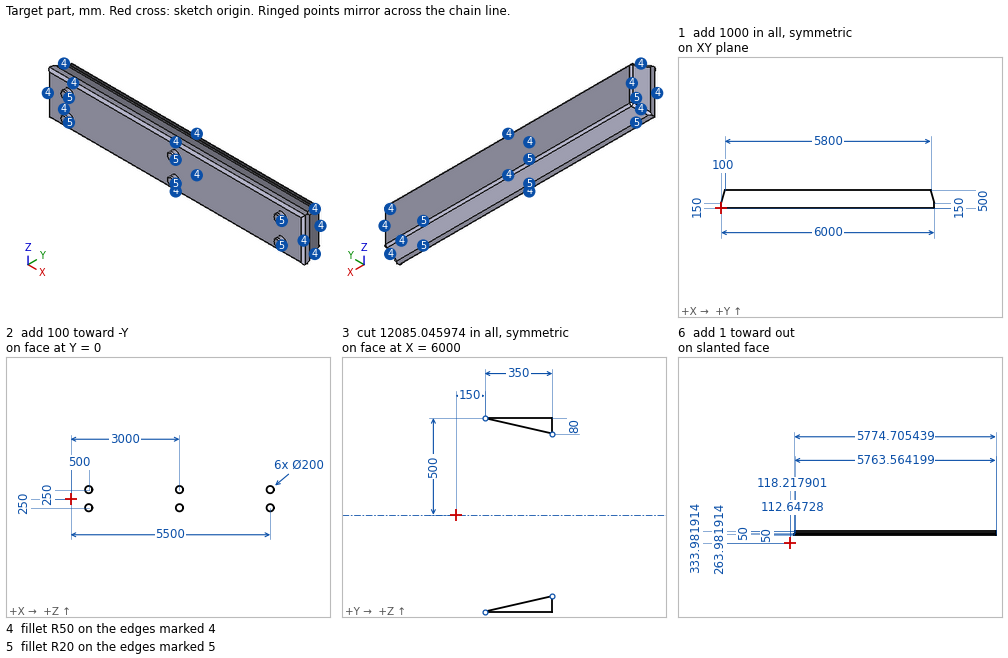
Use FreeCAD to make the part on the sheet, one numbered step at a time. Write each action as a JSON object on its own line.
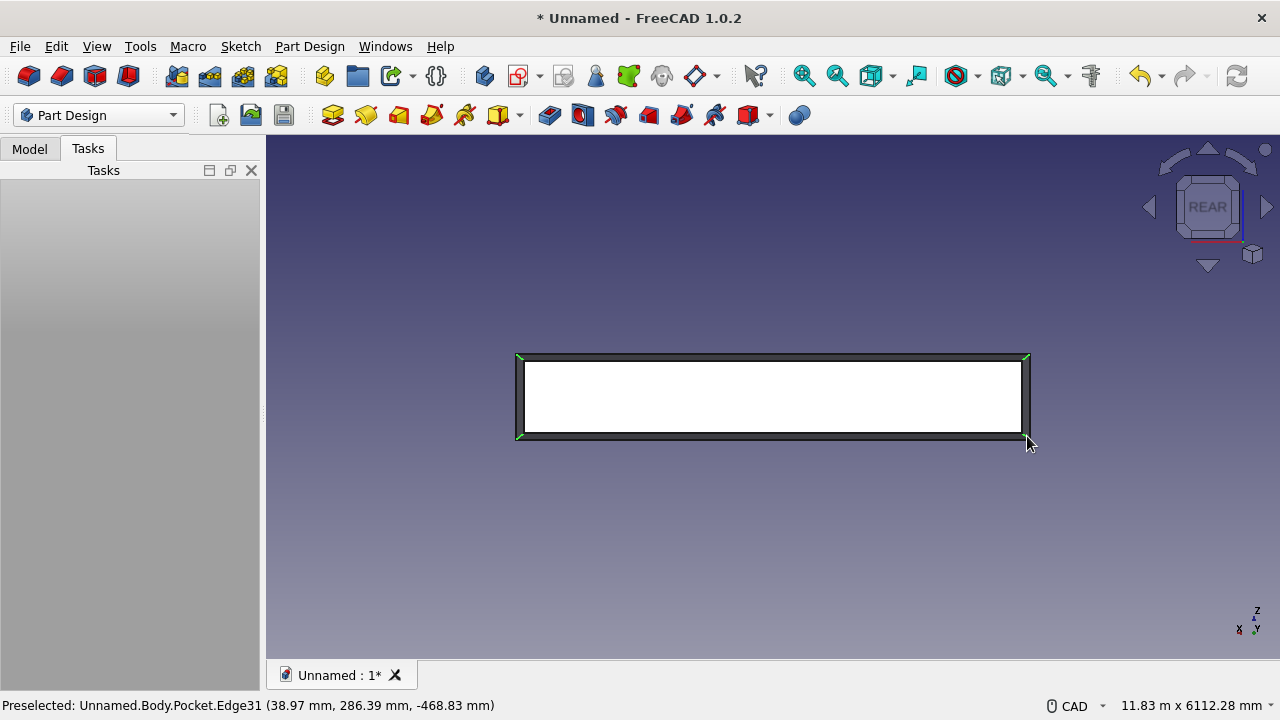
{"action": "left_click", "coordinate": [29, 76]}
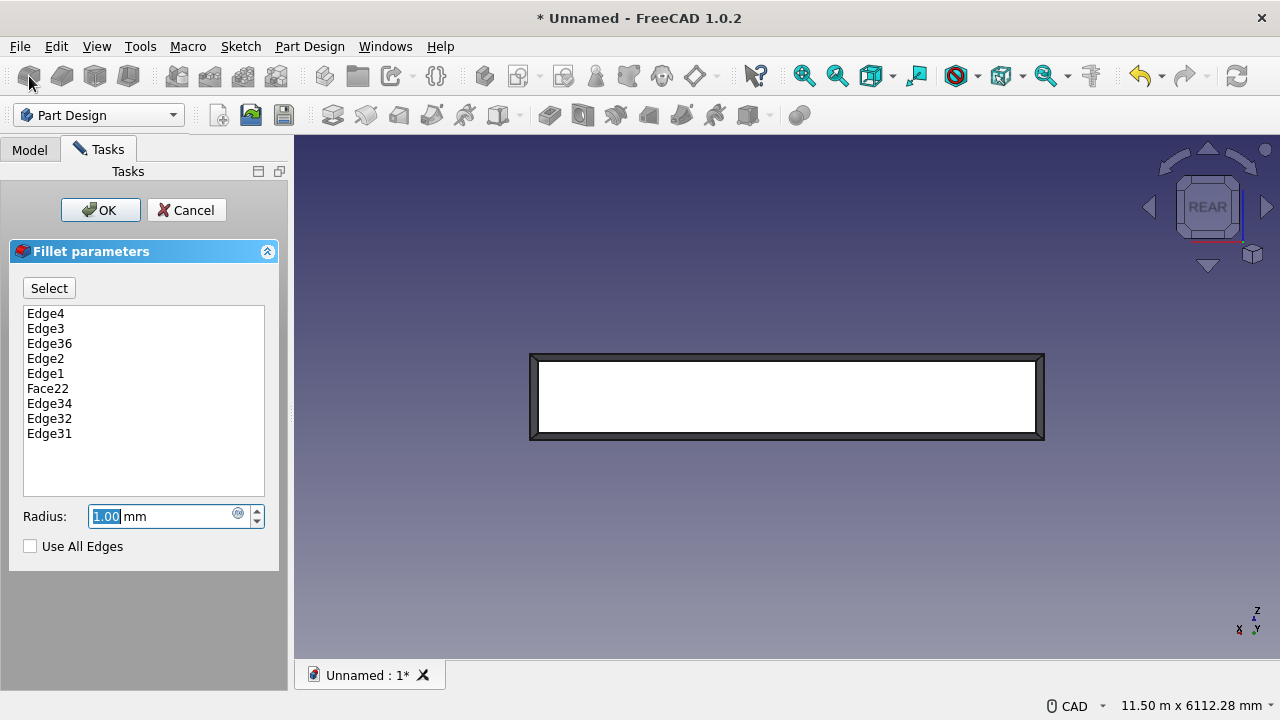
{"action": "type", "text": "50"}
{"action": "key", "text": "Tab"}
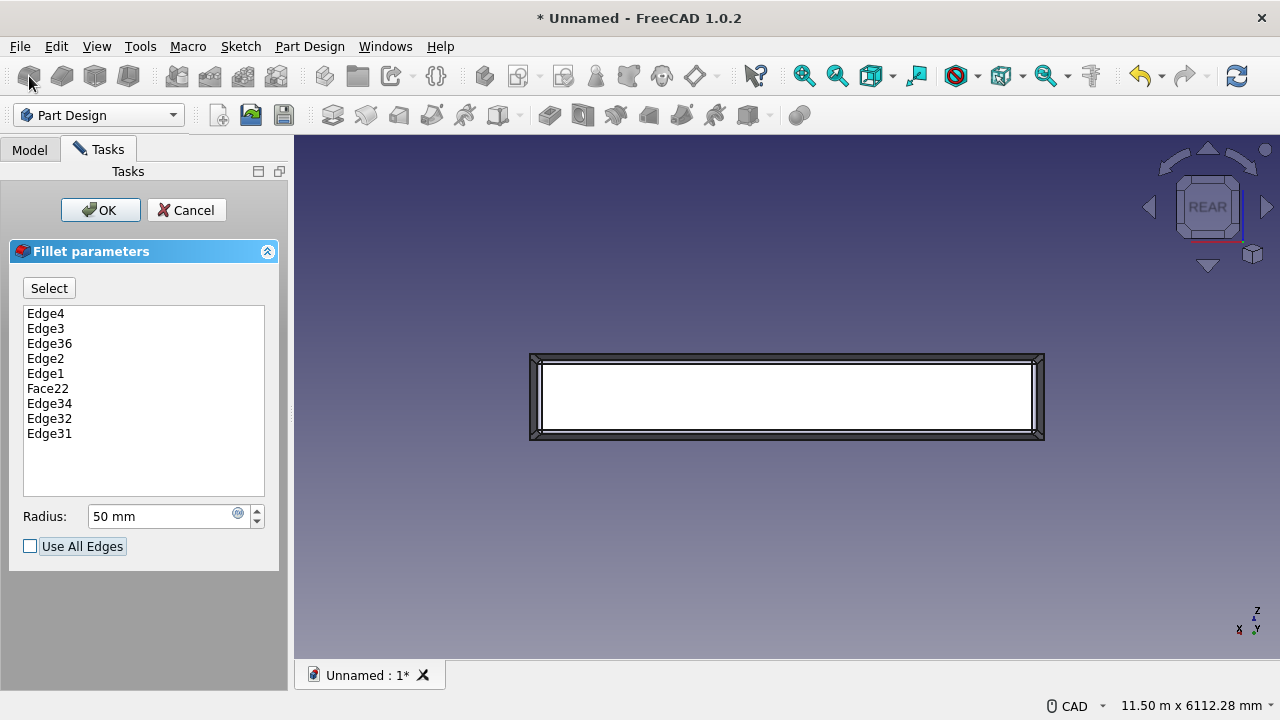
{"action": "left_click", "coordinate": [101, 210]}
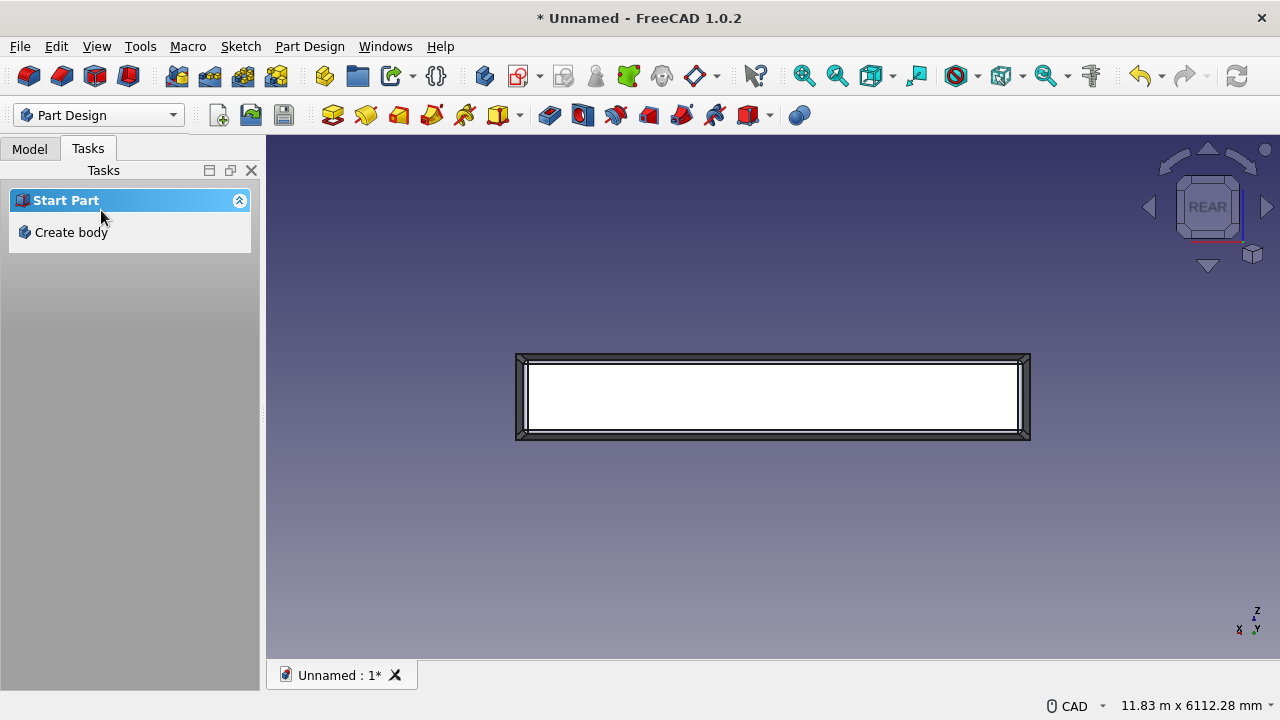
{"action": "key", "text": "0"}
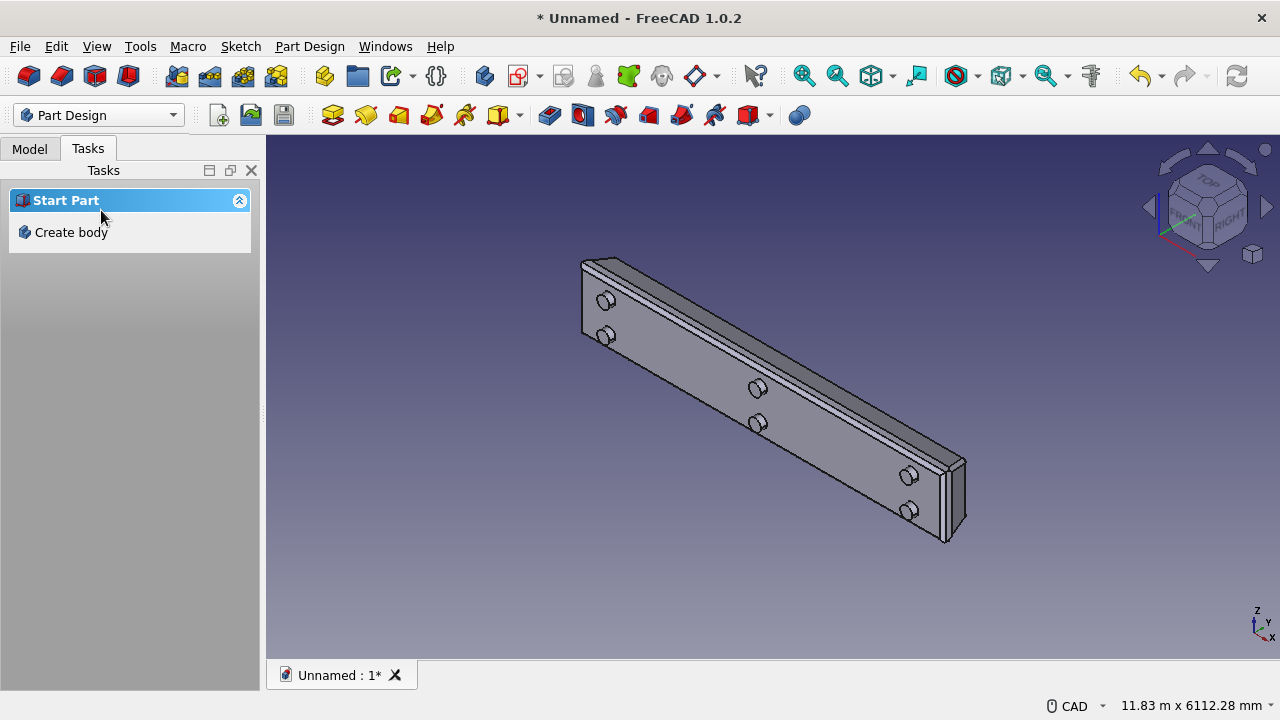
{"action": "left_click", "coordinate": [597, 298]}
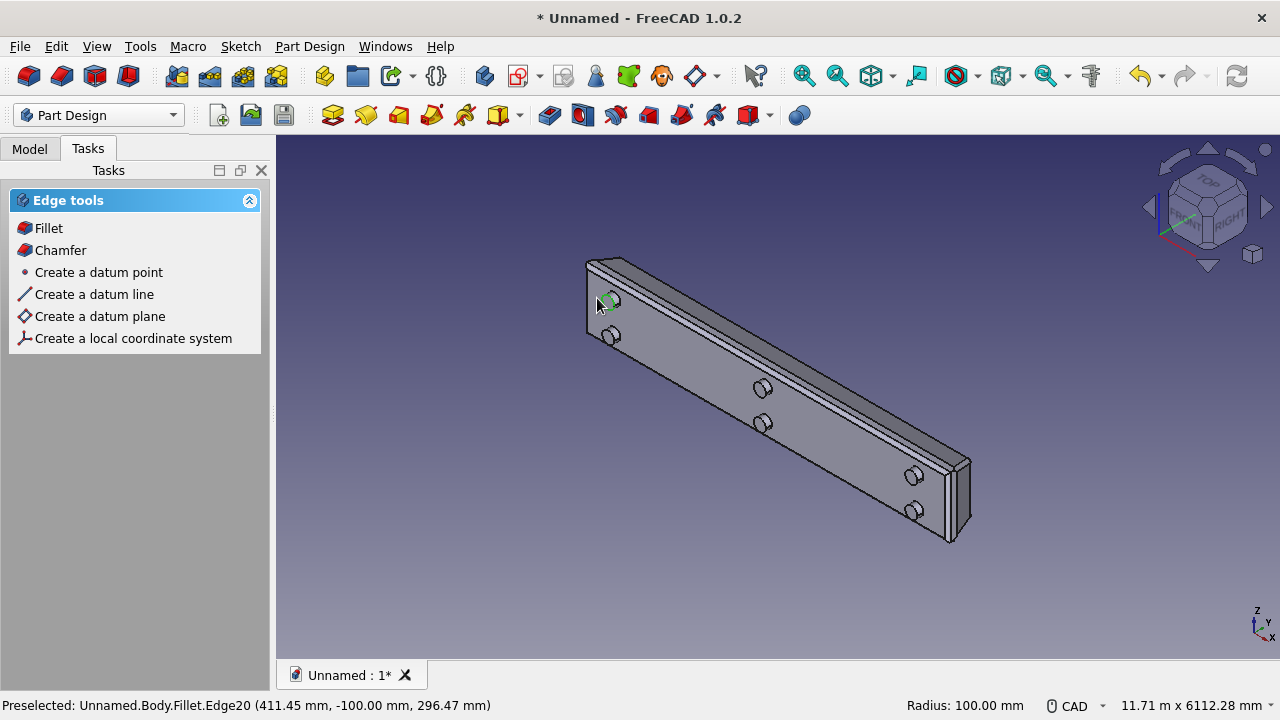
{"action": "left_click", "coordinate": [602, 333], "text": "ctrl"}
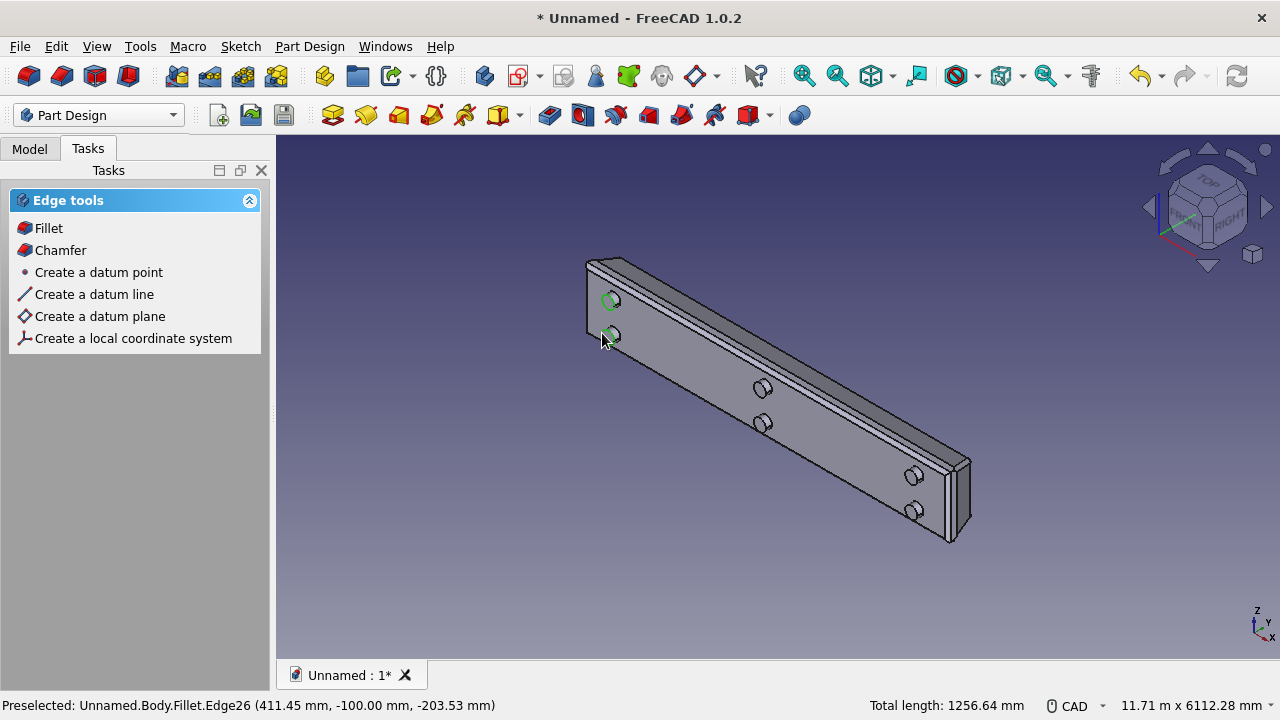
{"action": "left_click", "coordinate": [905, 508], "text": "ctrl"}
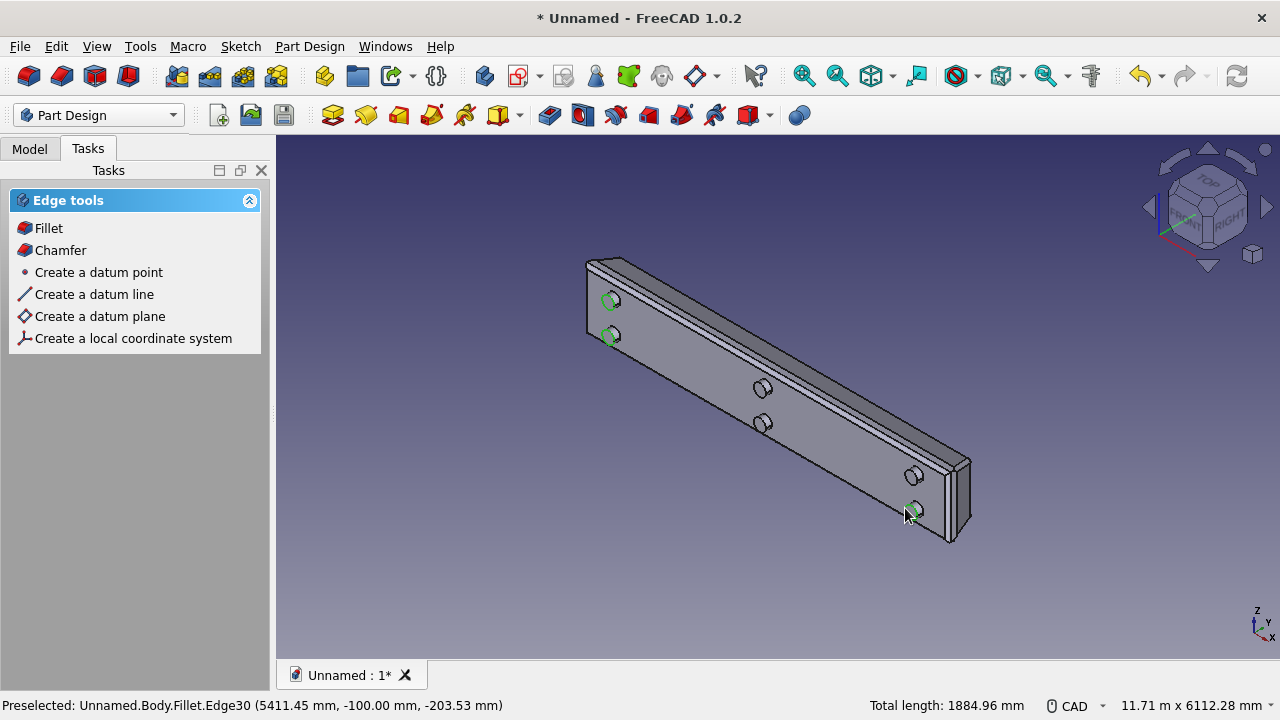
{"action": "left_click", "coordinate": [905, 473], "text": "ctrl"}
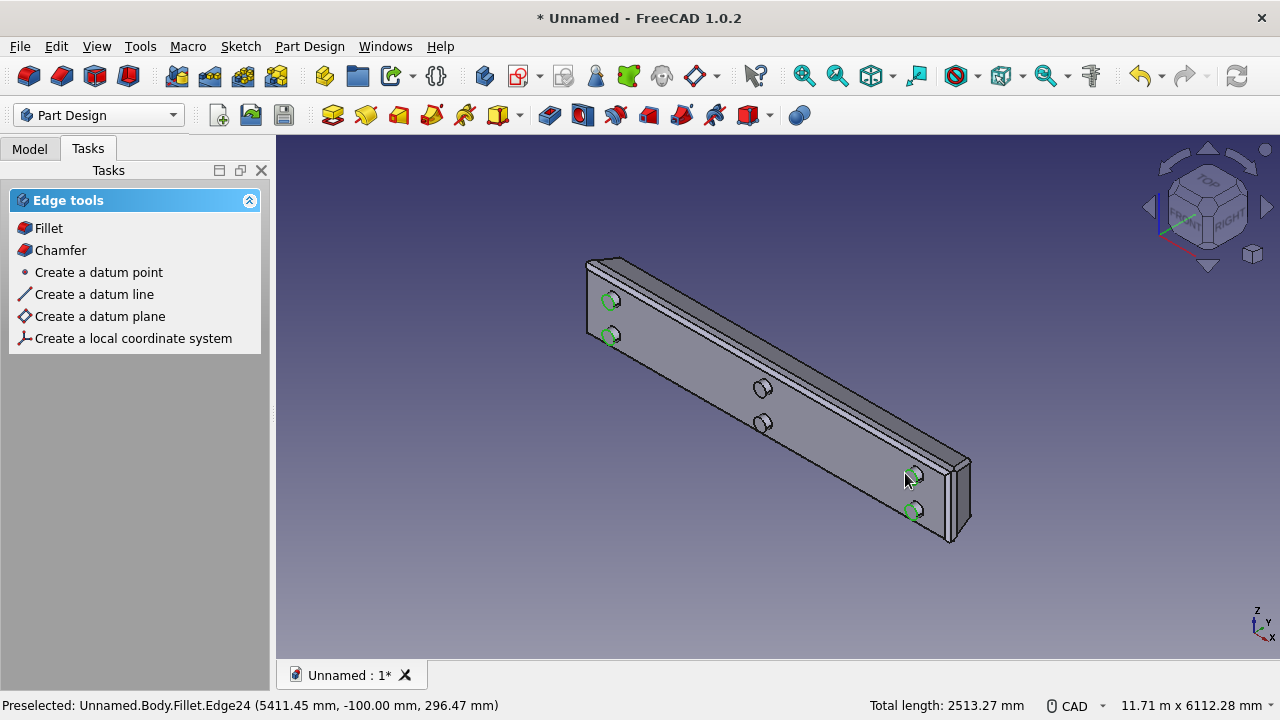
{"action": "left_click", "coordinate": [754, 386], "text": "ctrl"}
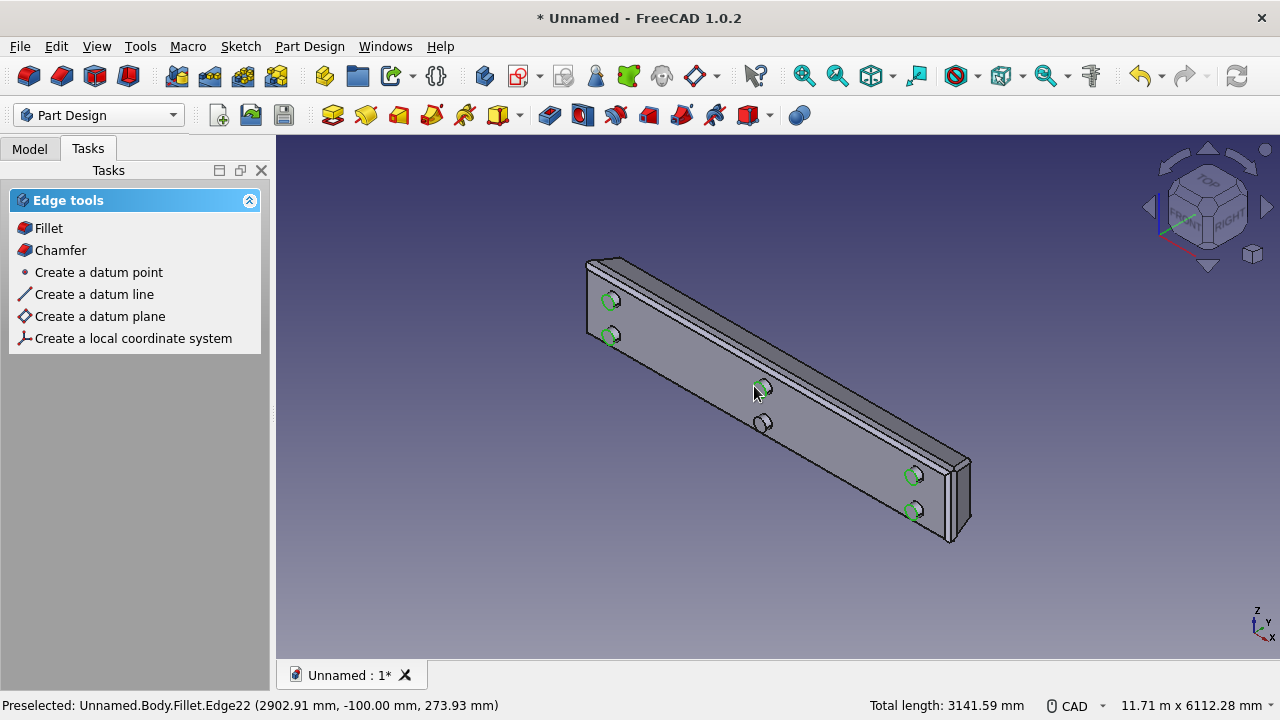
{"action": "left_click", "coordinate": [754, 420], "text": "ctrl"}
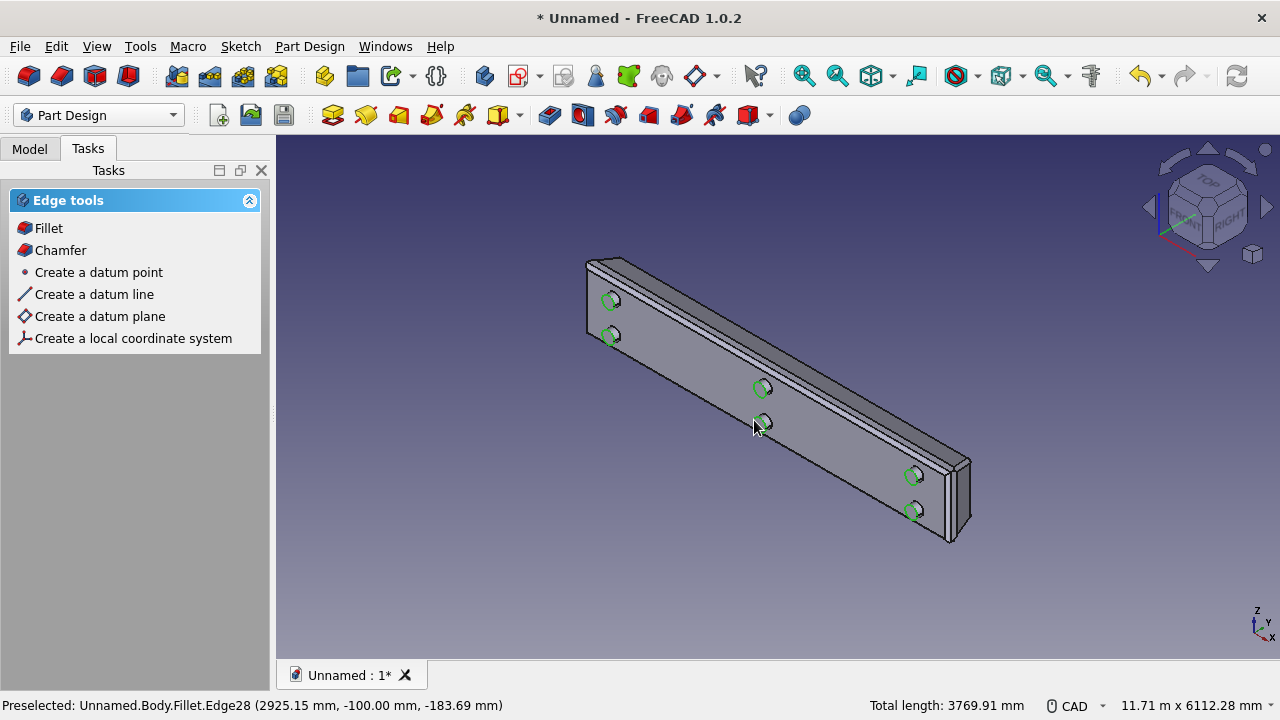
{"action": "left_click", "coordinate": [29, 76]}